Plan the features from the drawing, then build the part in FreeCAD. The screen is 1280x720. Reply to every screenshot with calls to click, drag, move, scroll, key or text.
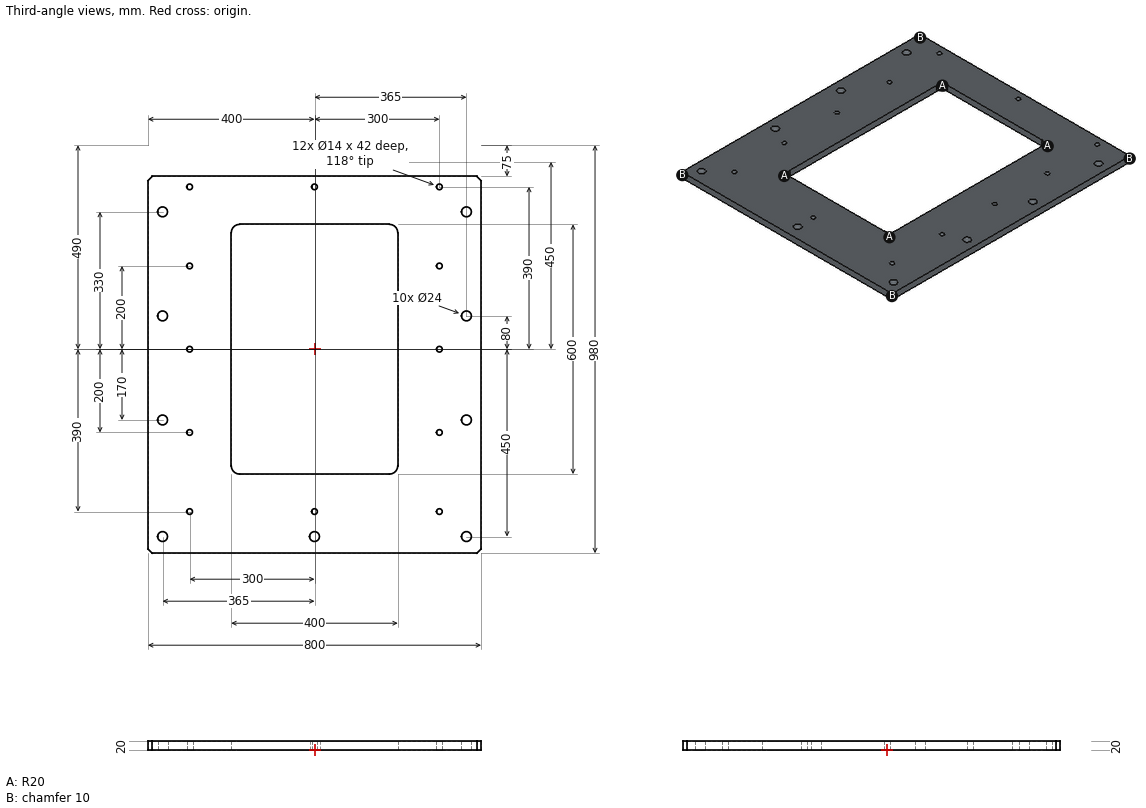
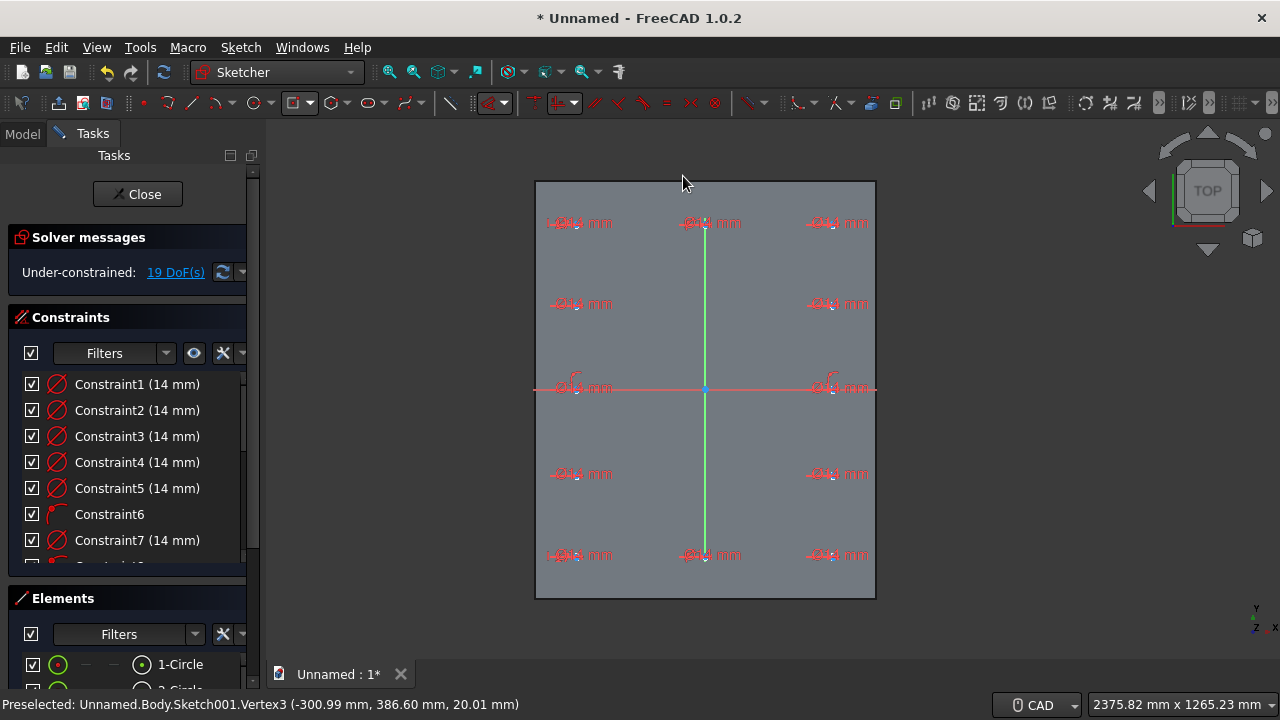
click(833, 225)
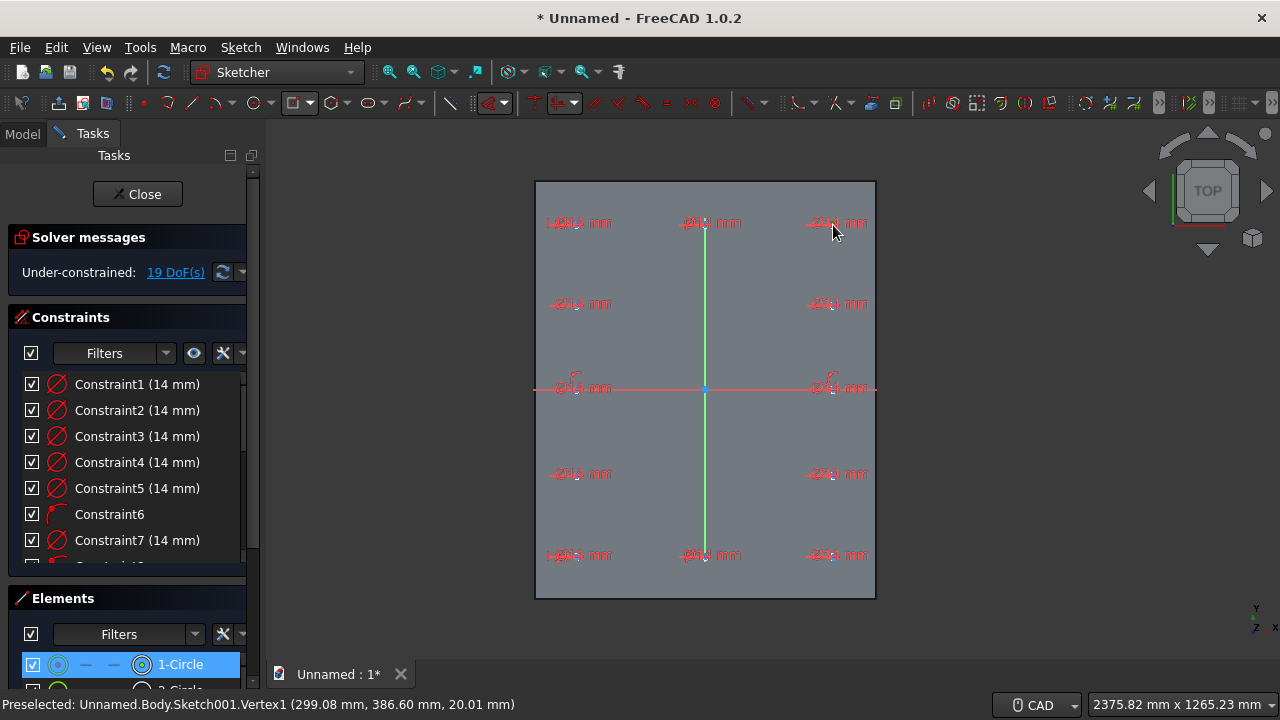
click(577, 225)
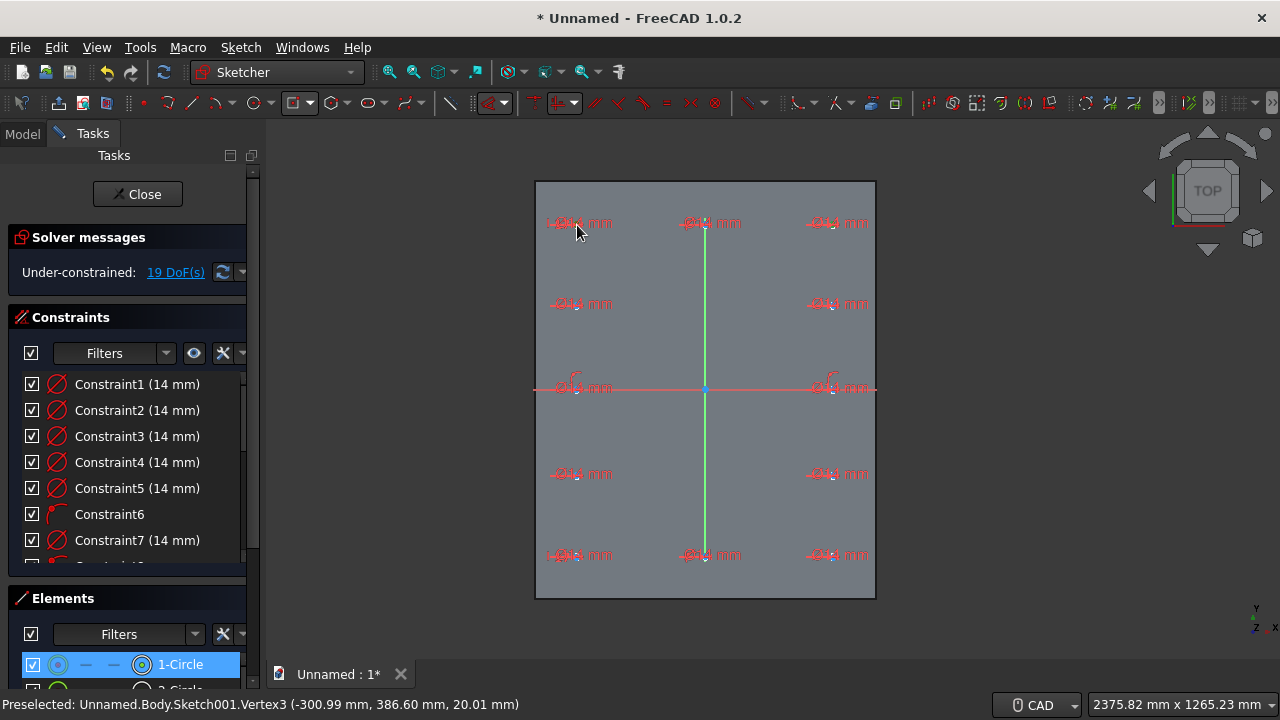
click(576, 104)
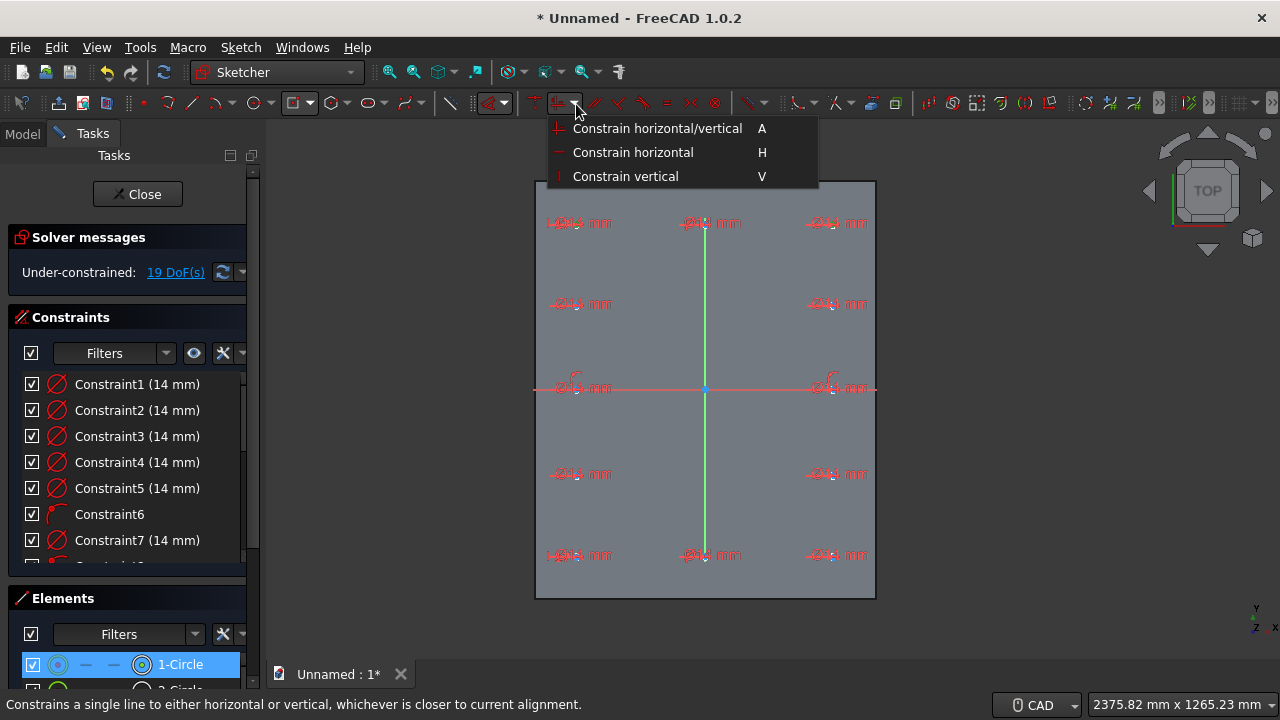
click(683, 152)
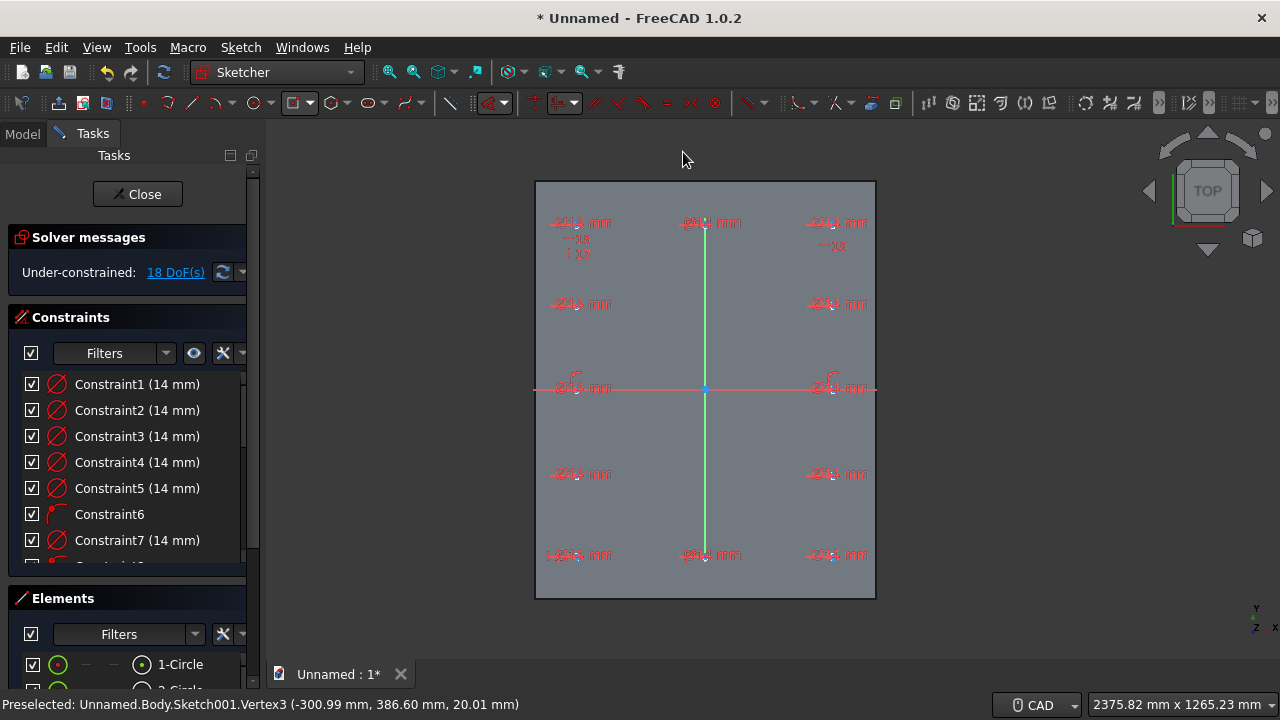
click(833, 225)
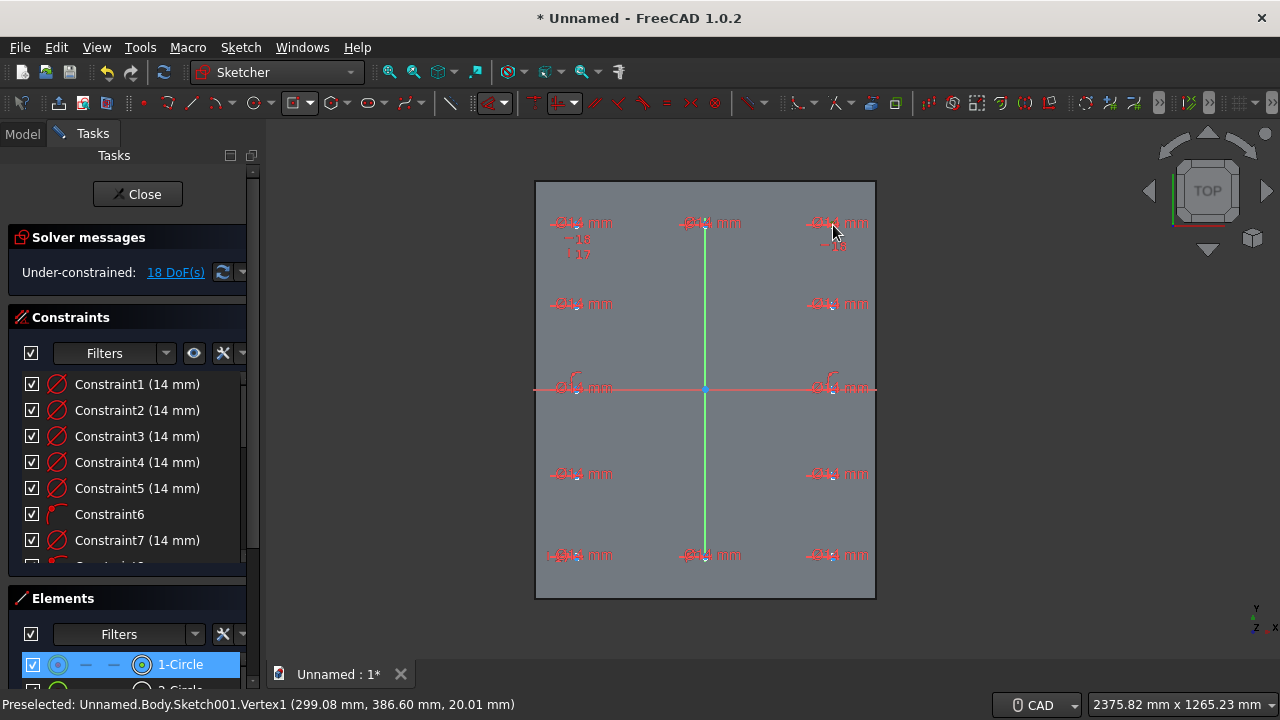
click(833, 557)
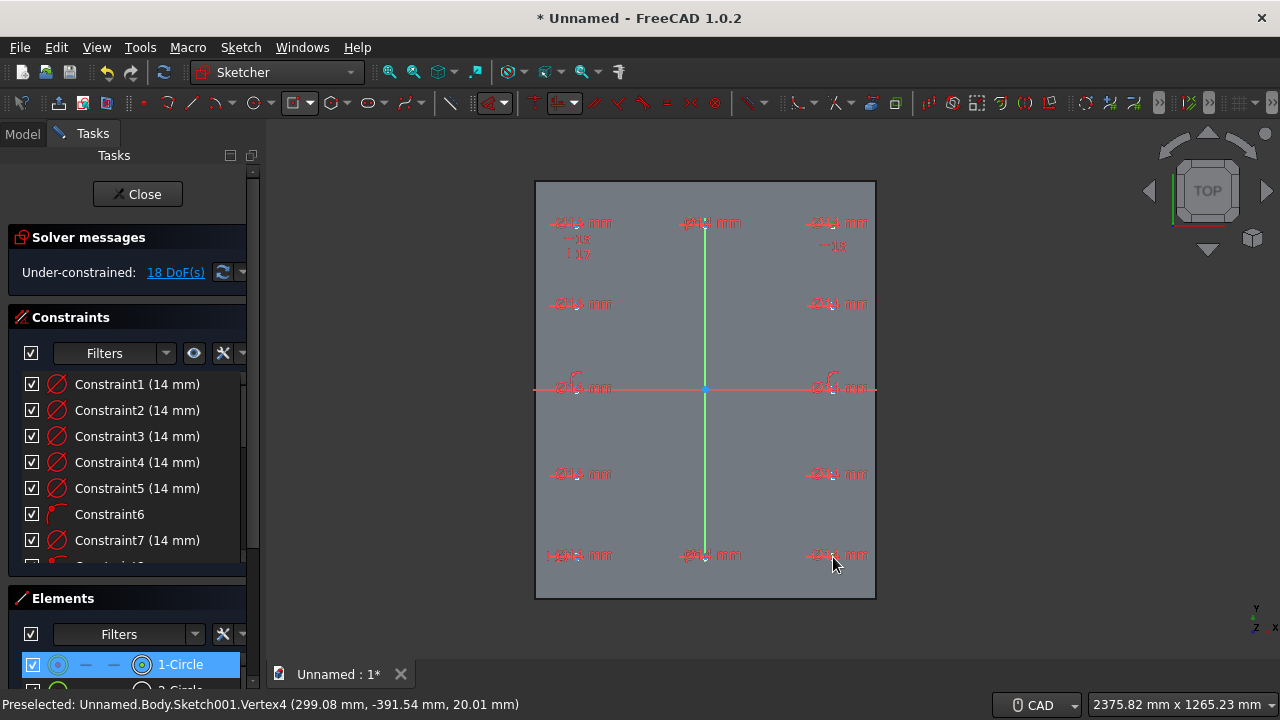
key(v)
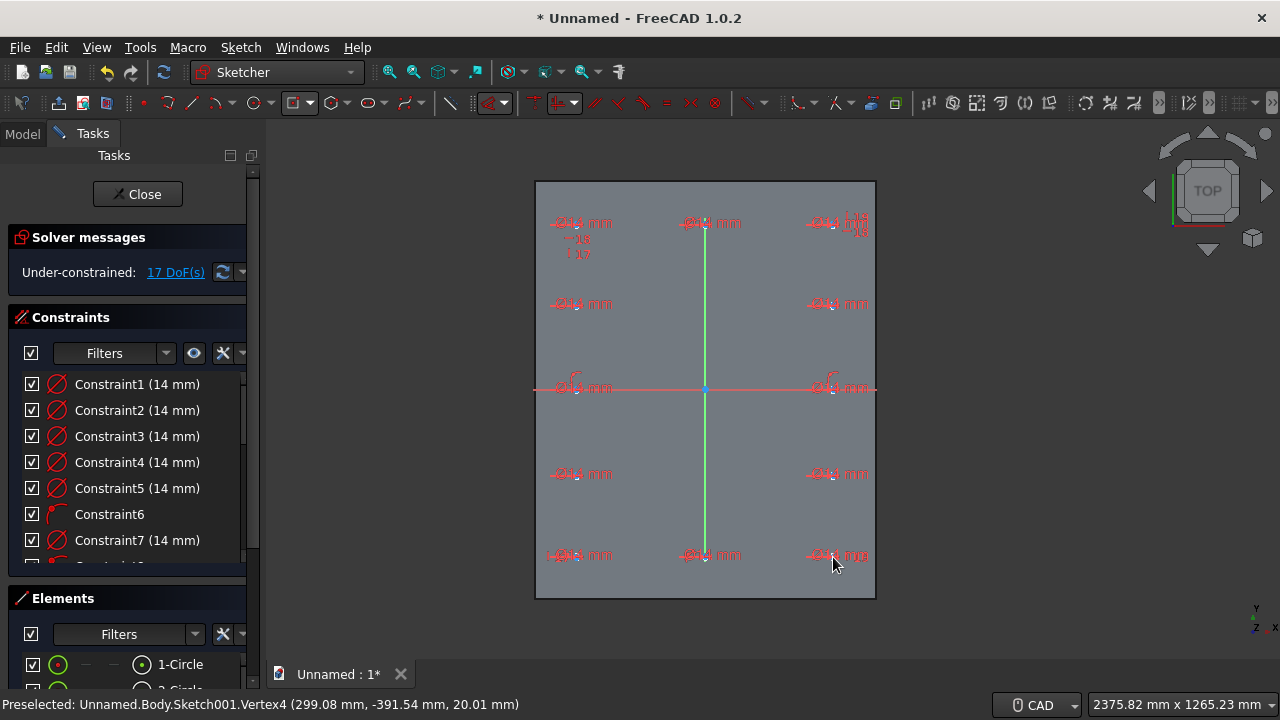
click(577, 557)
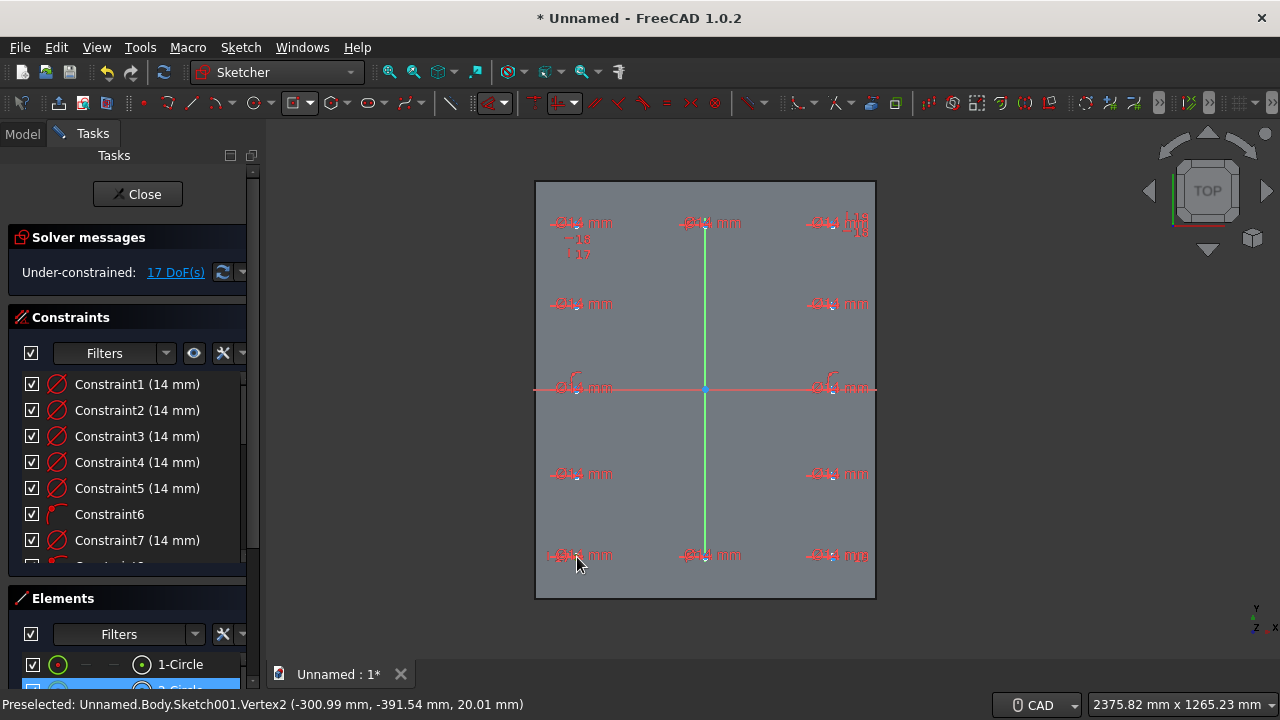
click(833, 557)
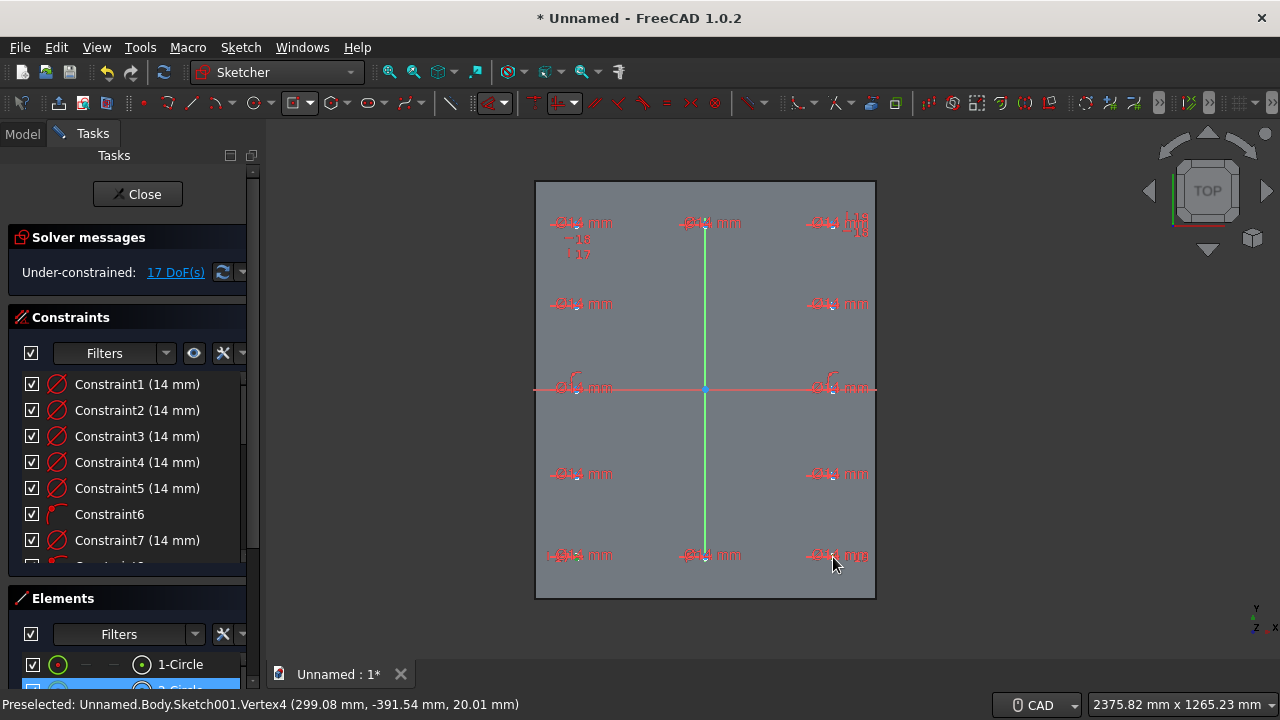
click(576, 104)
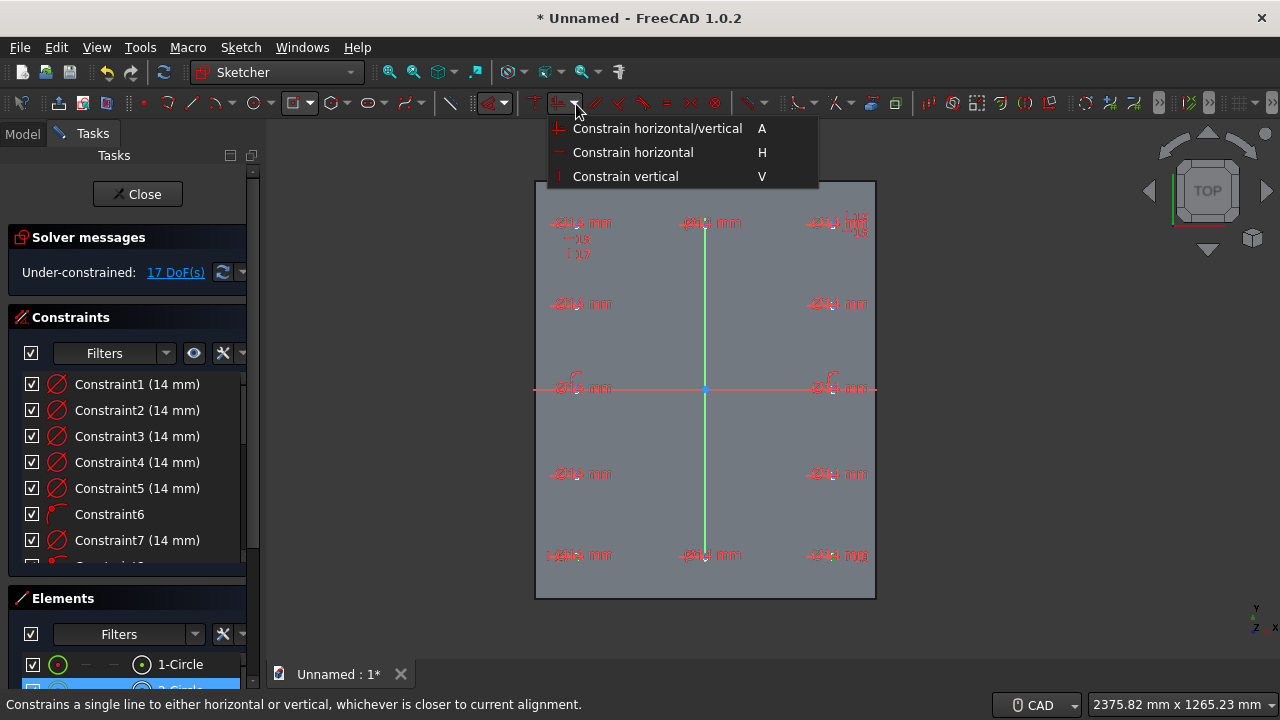
click(683, 152)